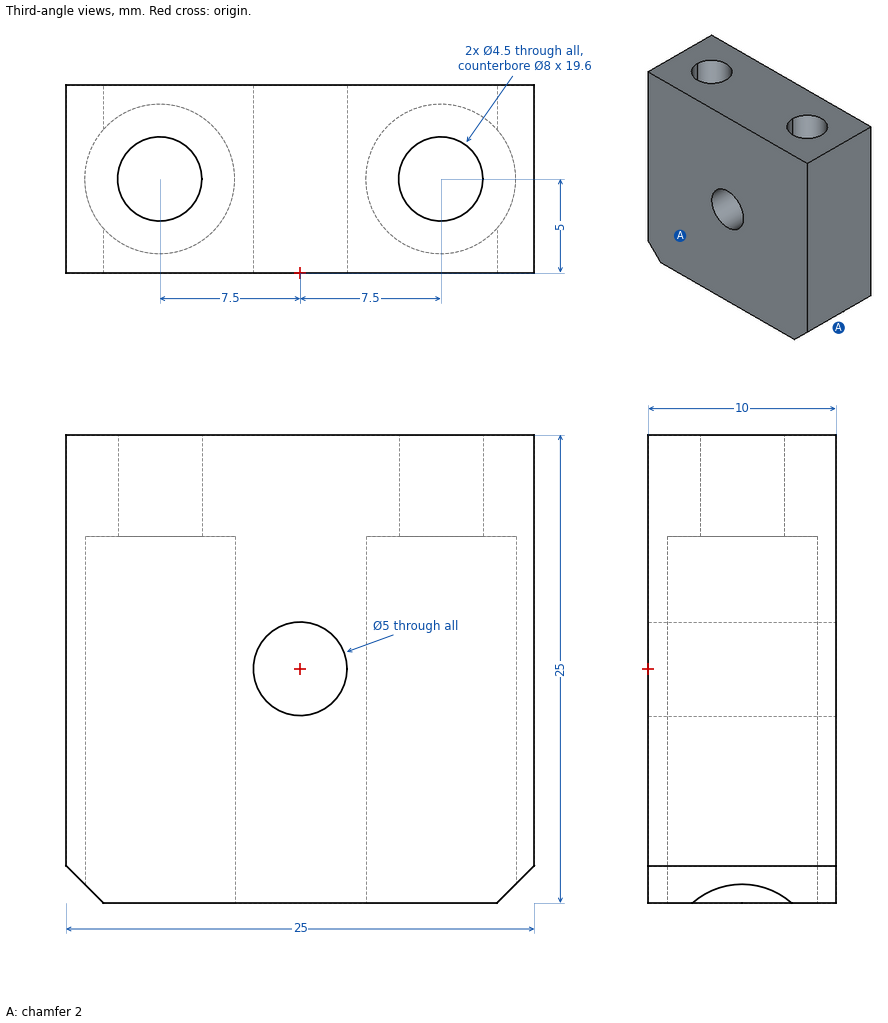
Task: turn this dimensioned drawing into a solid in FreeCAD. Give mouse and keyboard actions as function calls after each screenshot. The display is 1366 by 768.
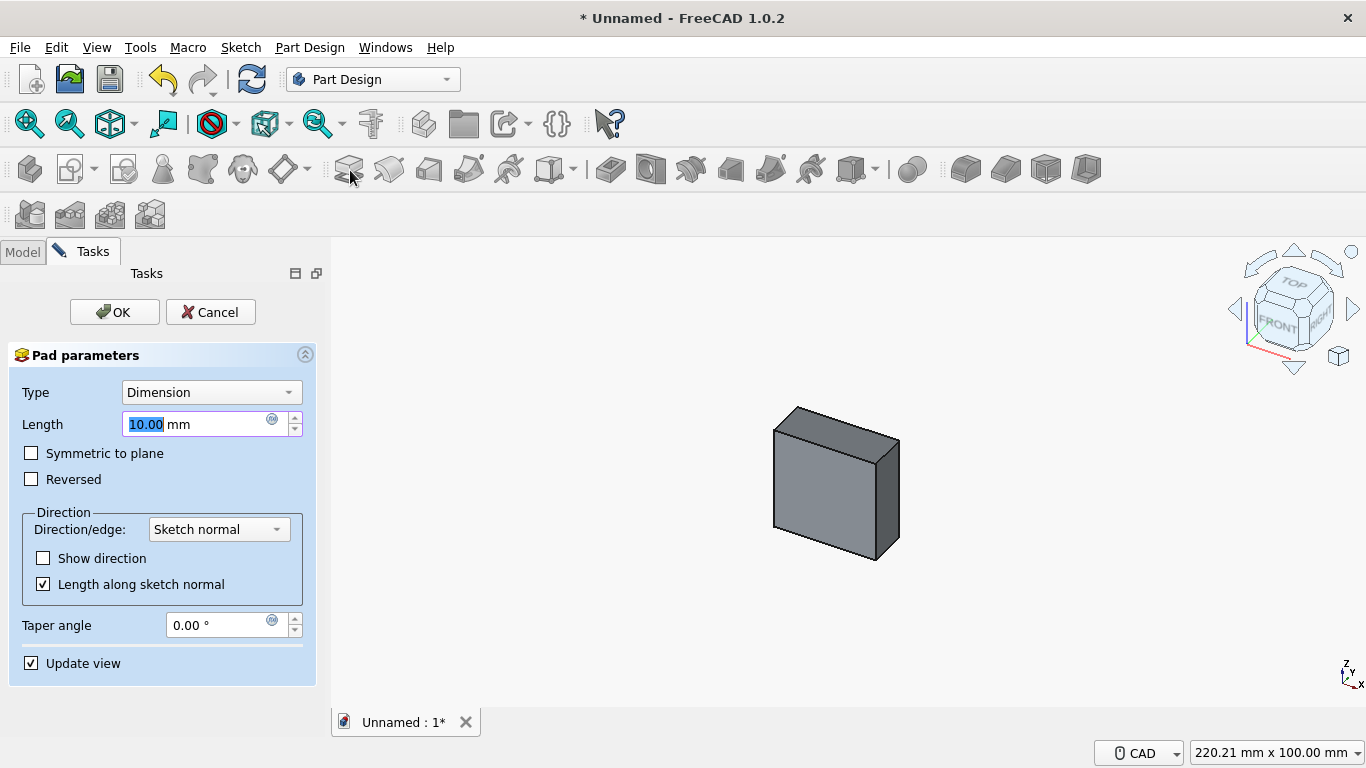
text(10)
key(Tab)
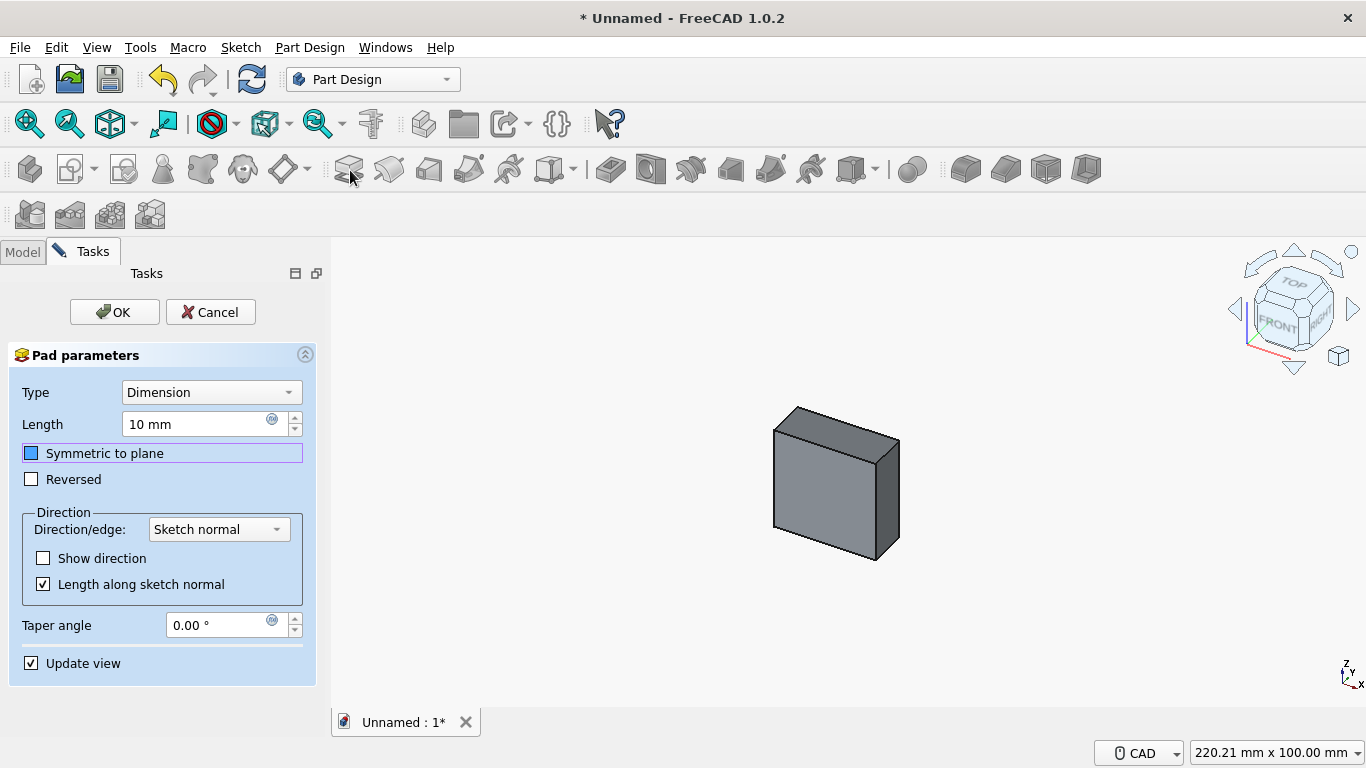
click(30, 479)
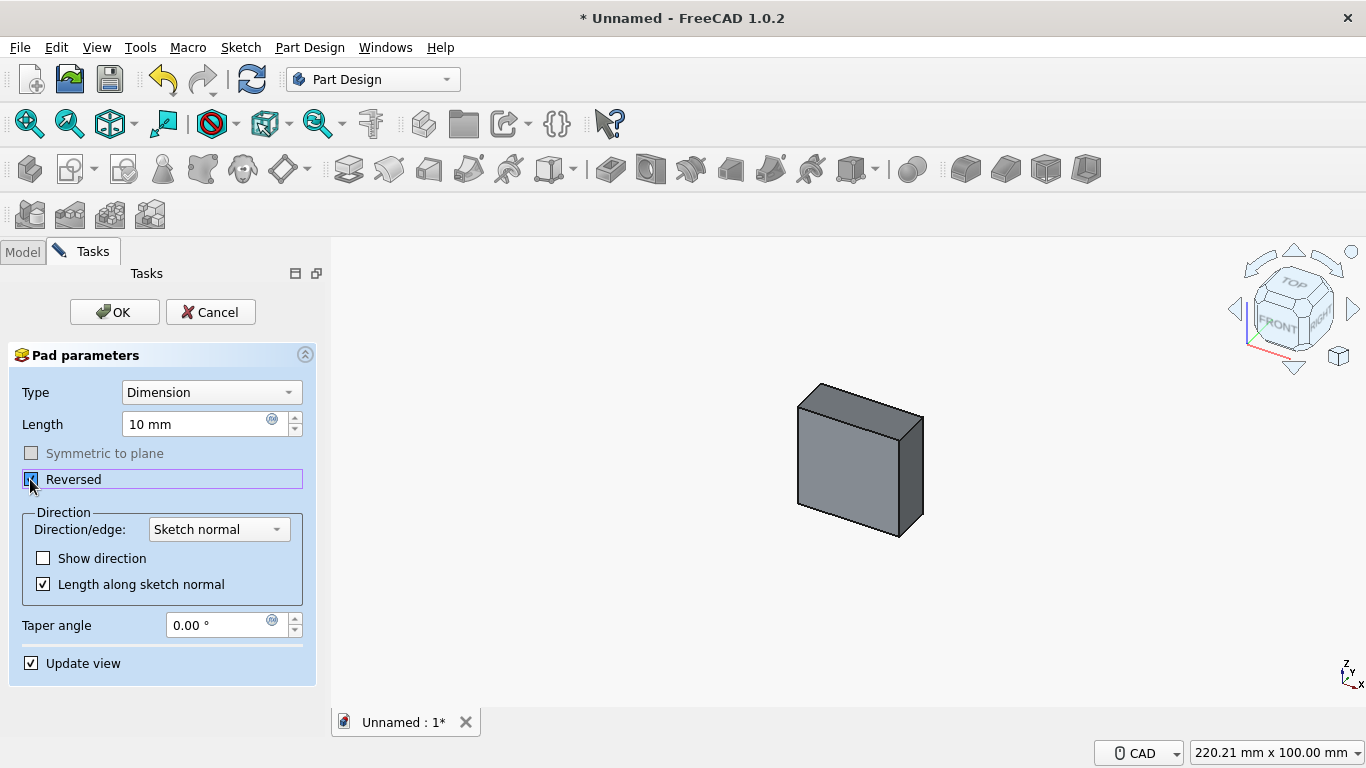
click(115, 312)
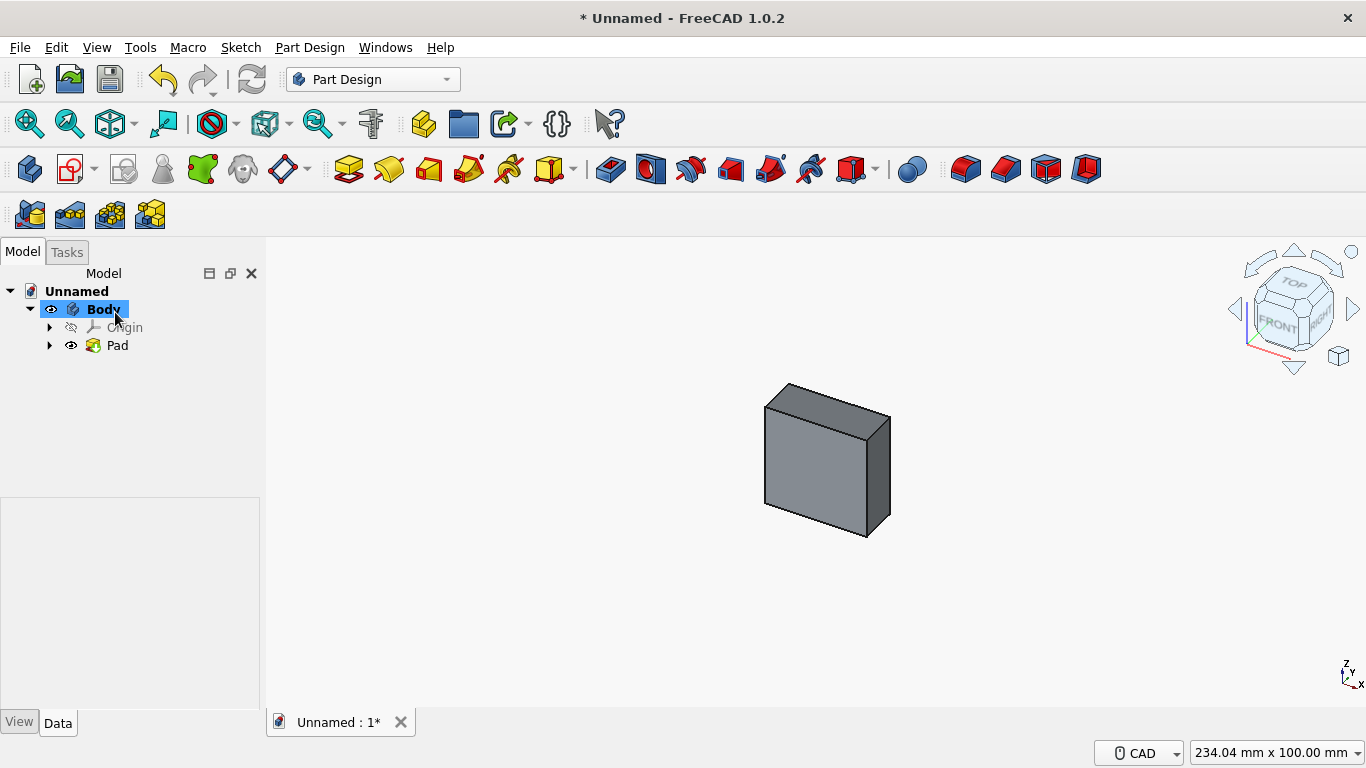
key(v)
key(f)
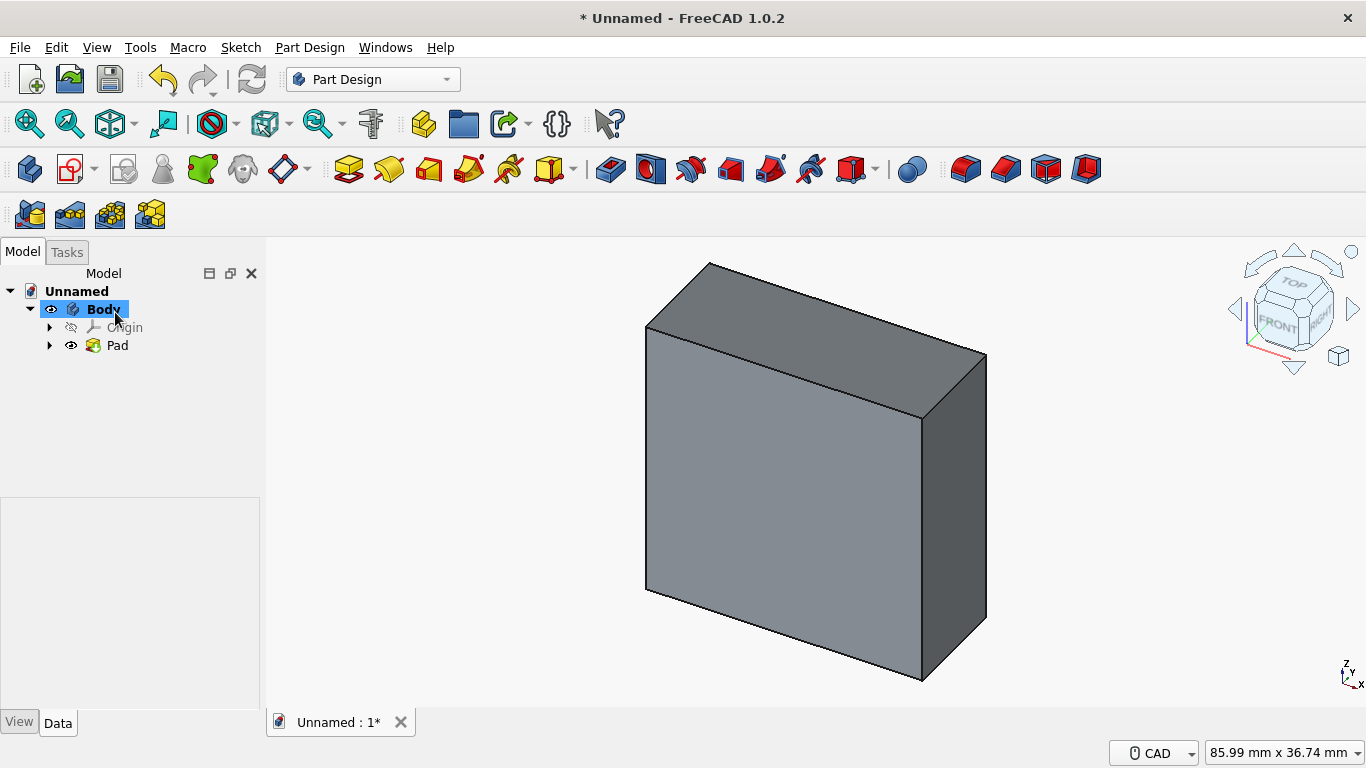
key(0)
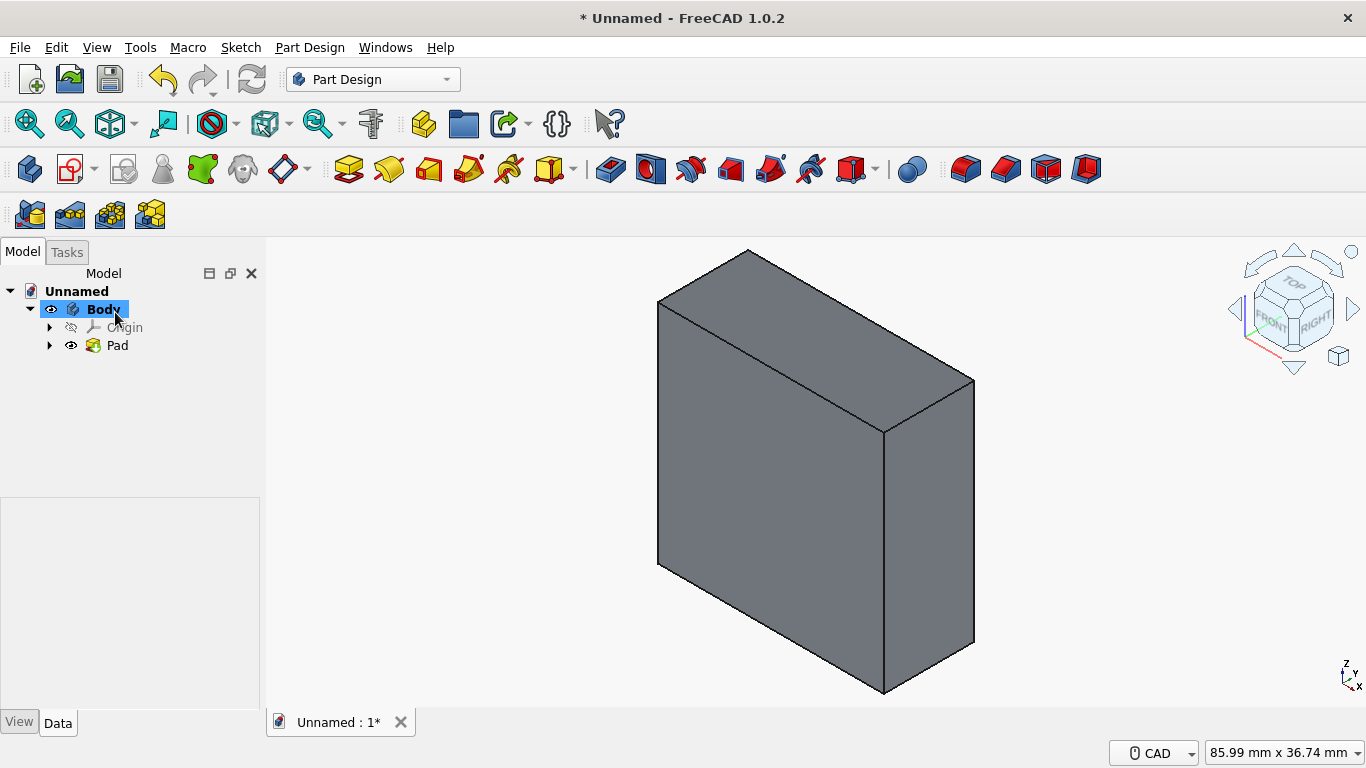
key(2)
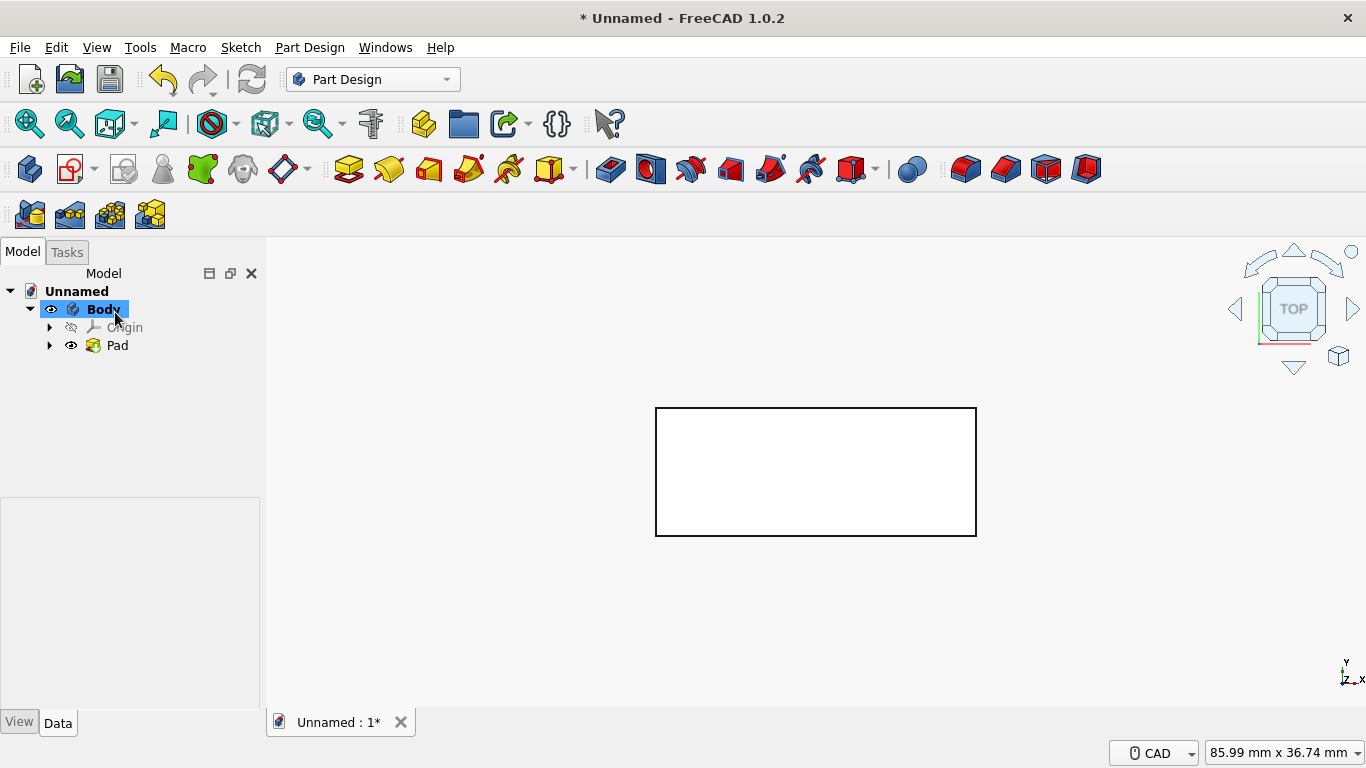
key(v)
key(f)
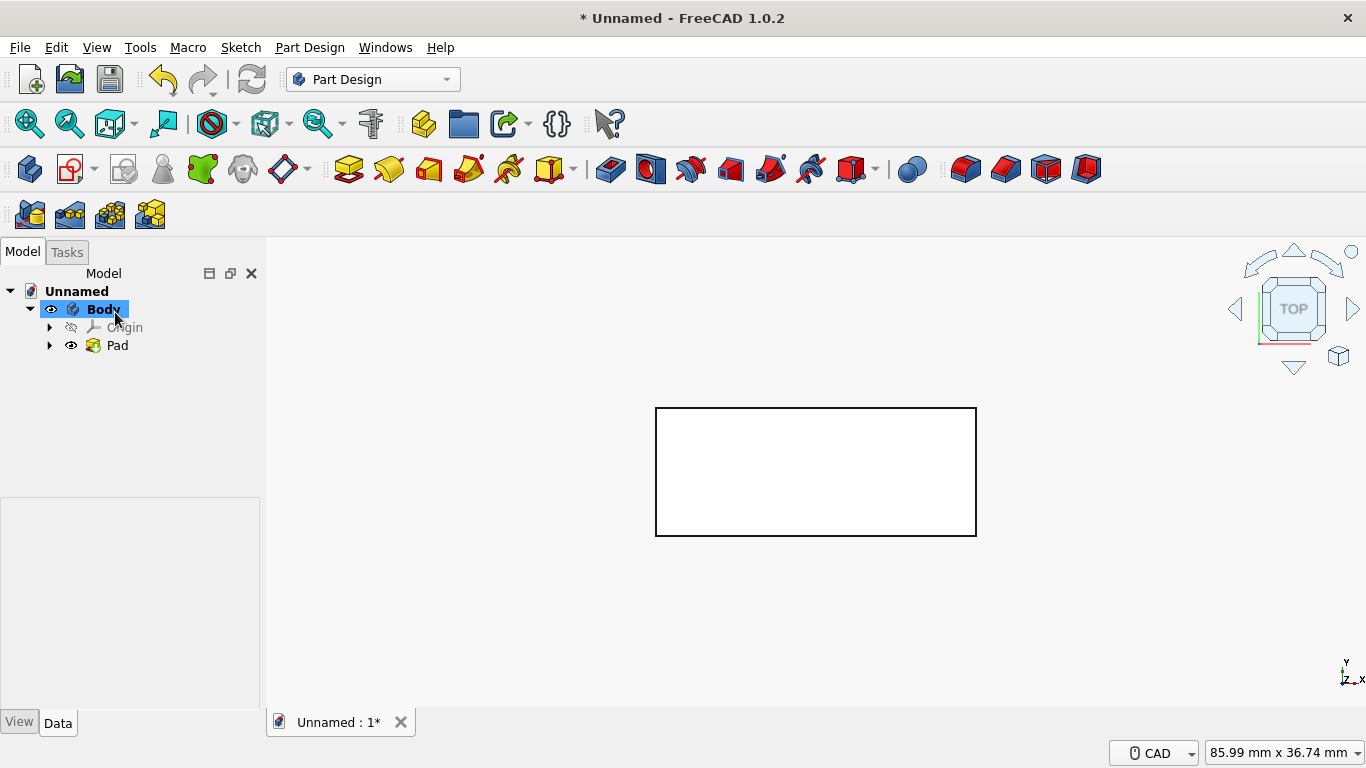
key(1)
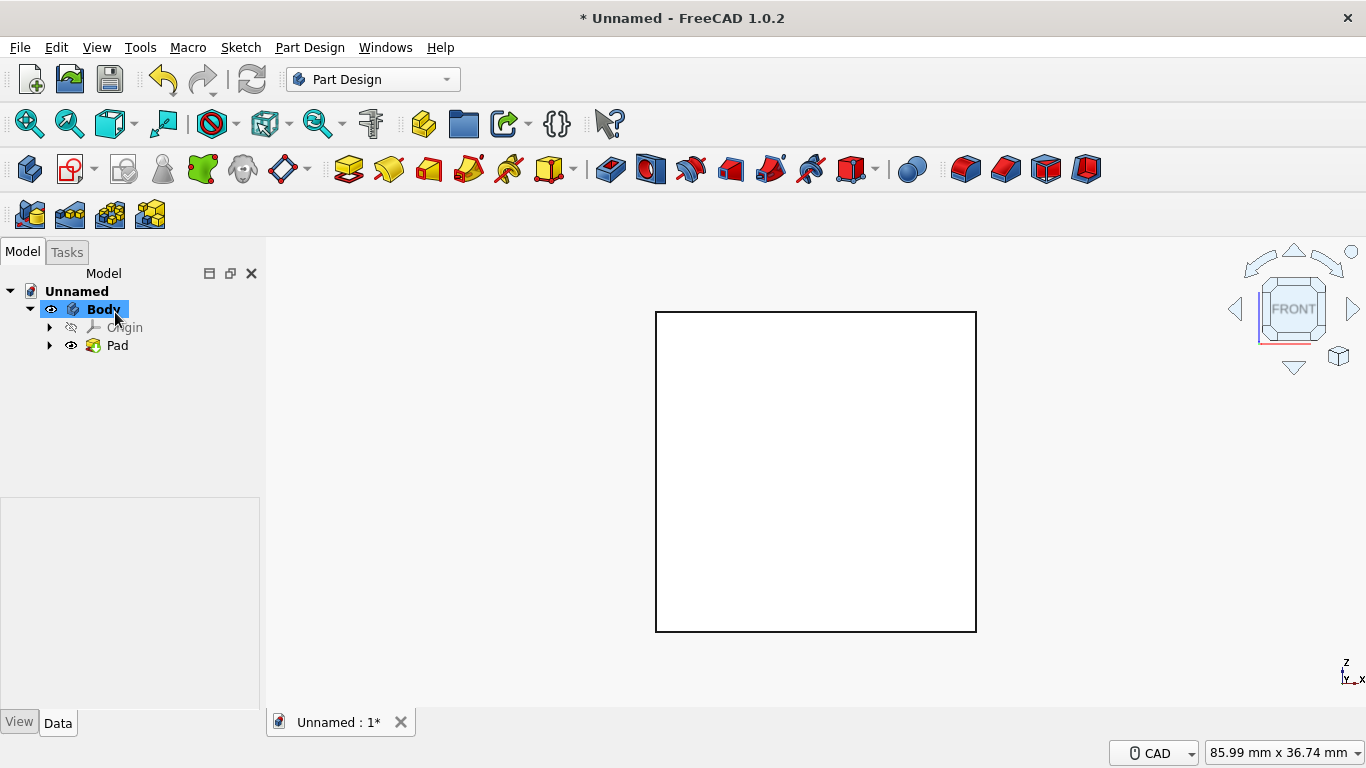
key(3)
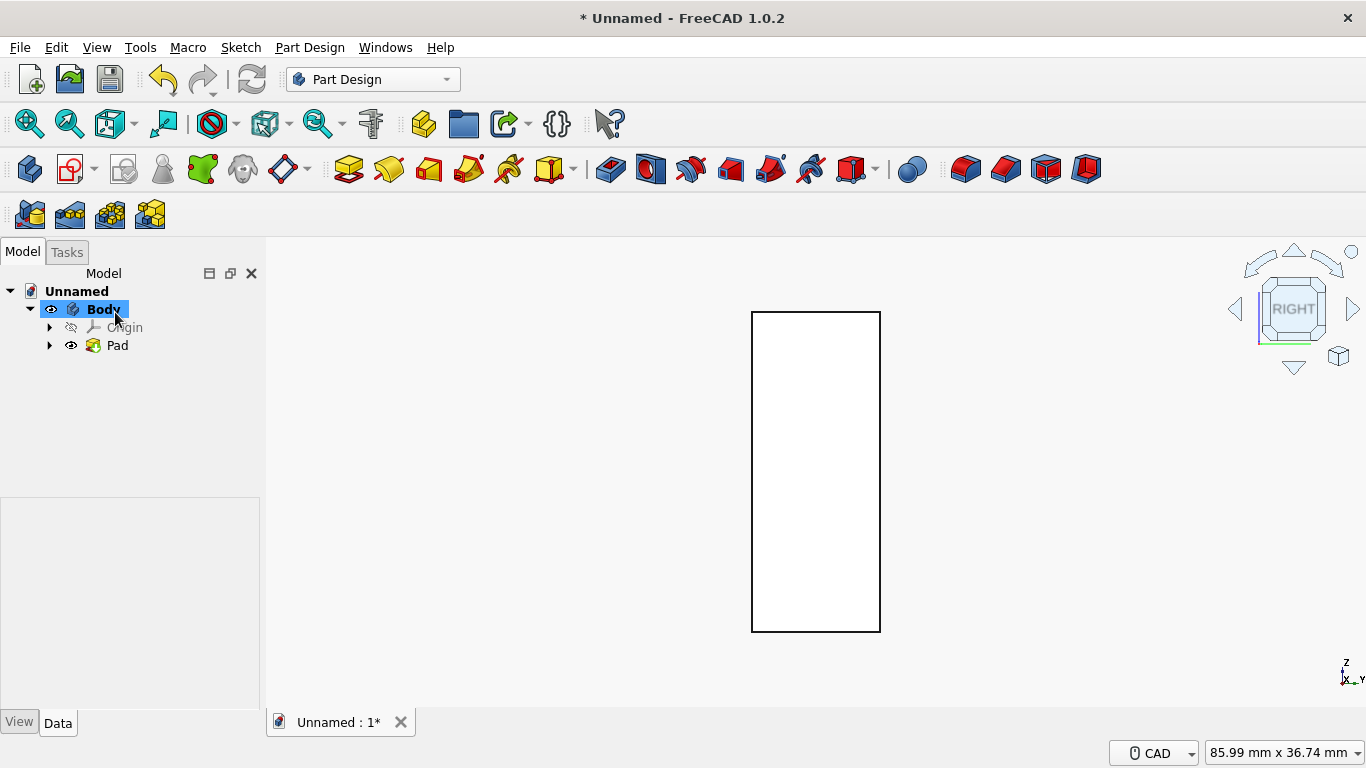
click(816, 631)